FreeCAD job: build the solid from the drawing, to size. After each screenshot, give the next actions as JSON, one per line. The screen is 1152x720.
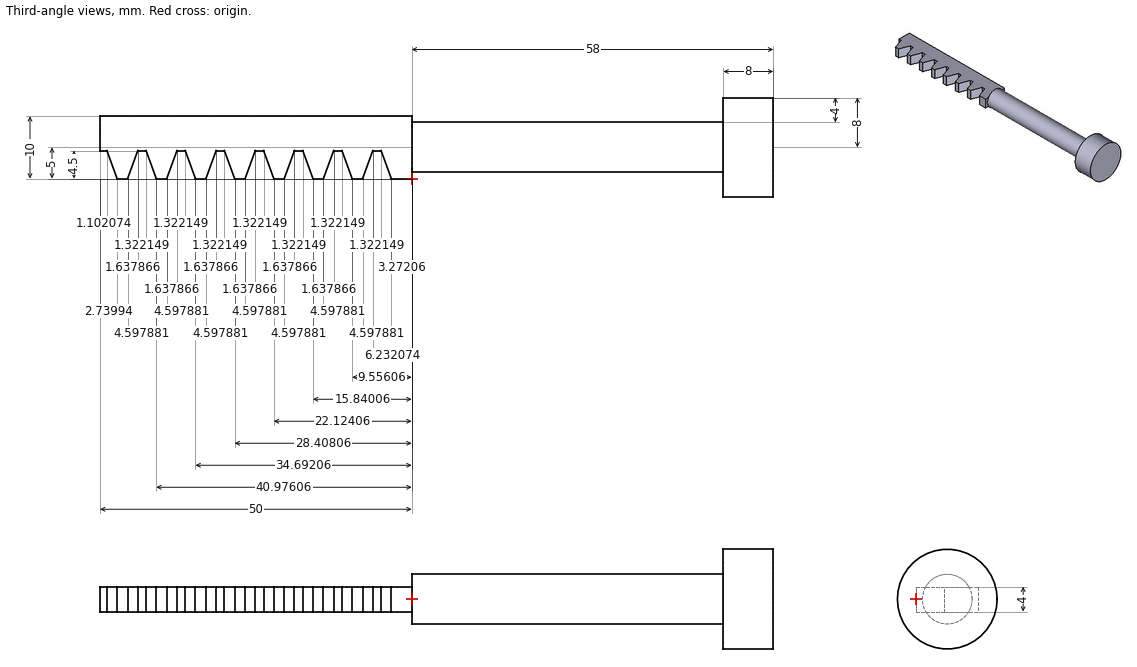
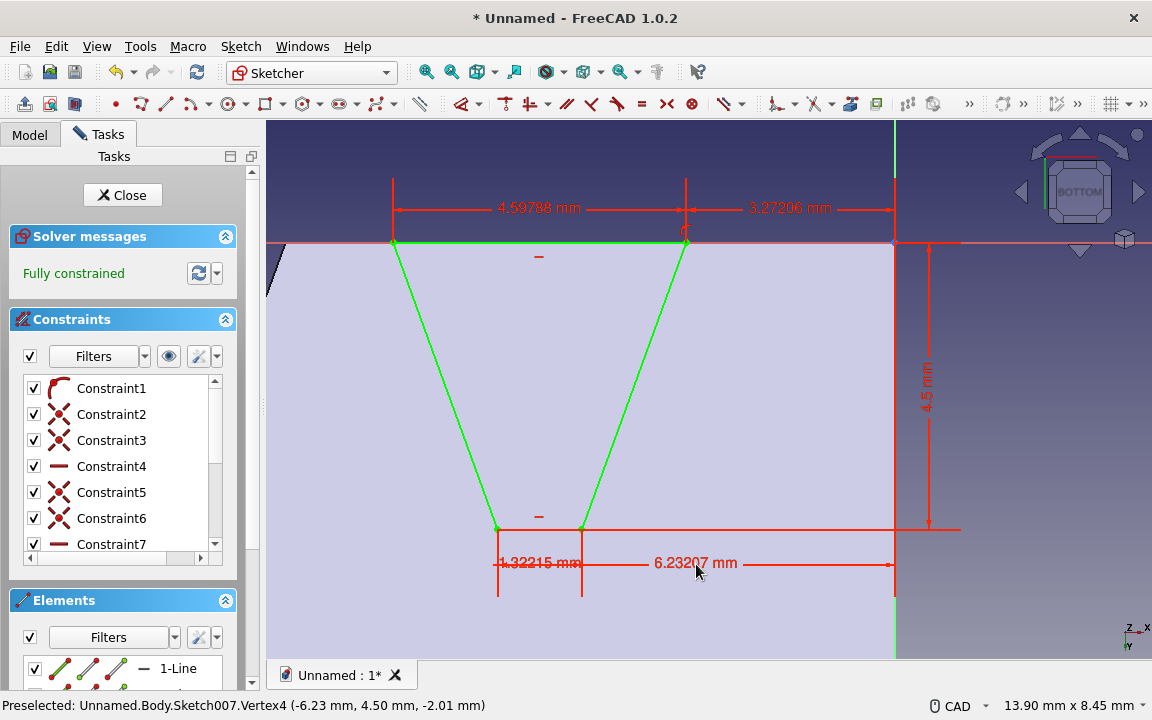
{"action": "left_click", "coordinate": [123, 195]}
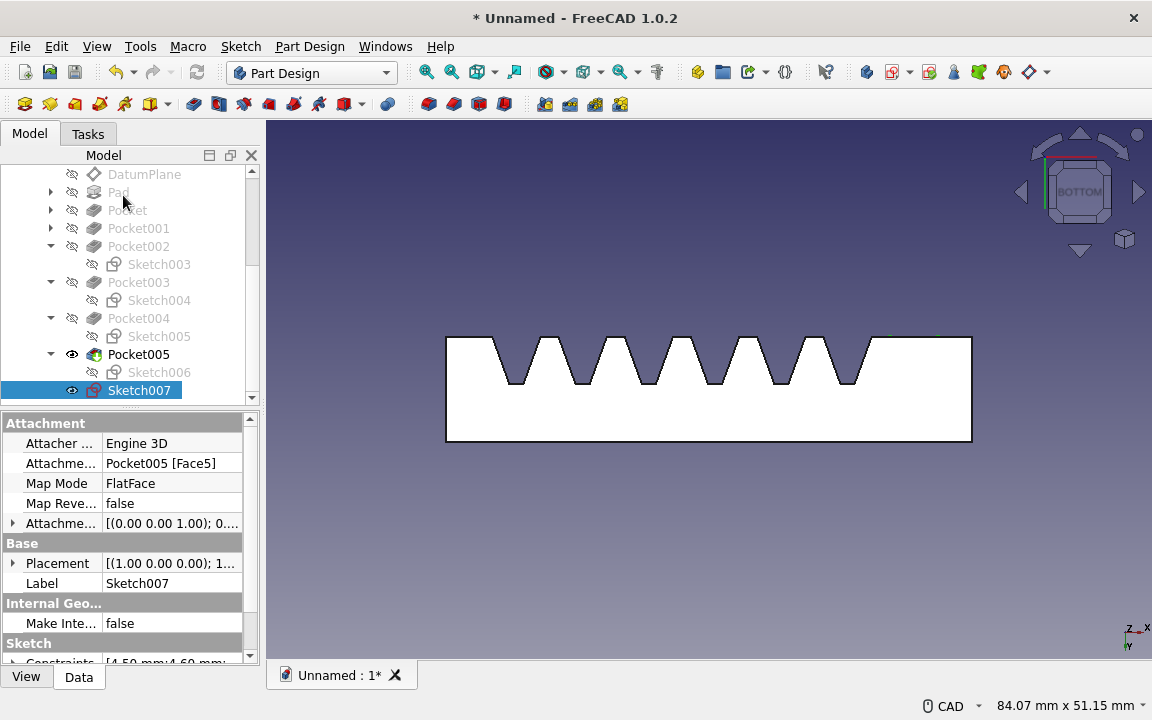
{"action": "left_click", "coordinate": [194, 104]}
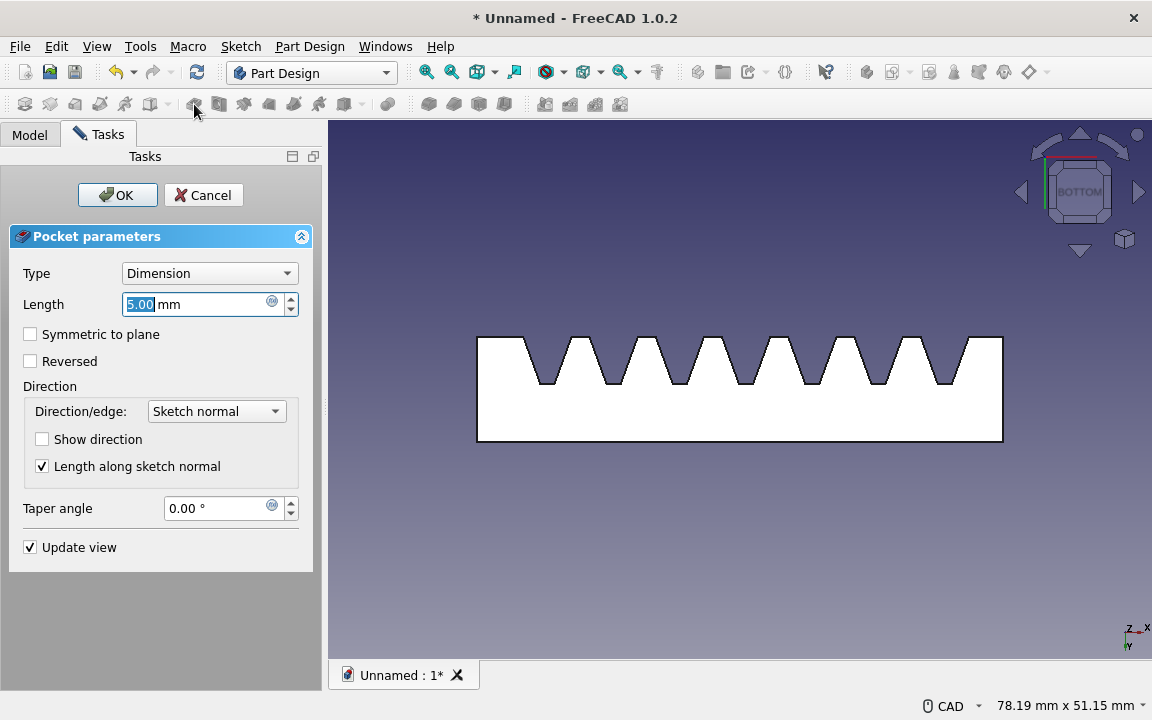
{"action": "left_click", "coordinate": [210, 274]}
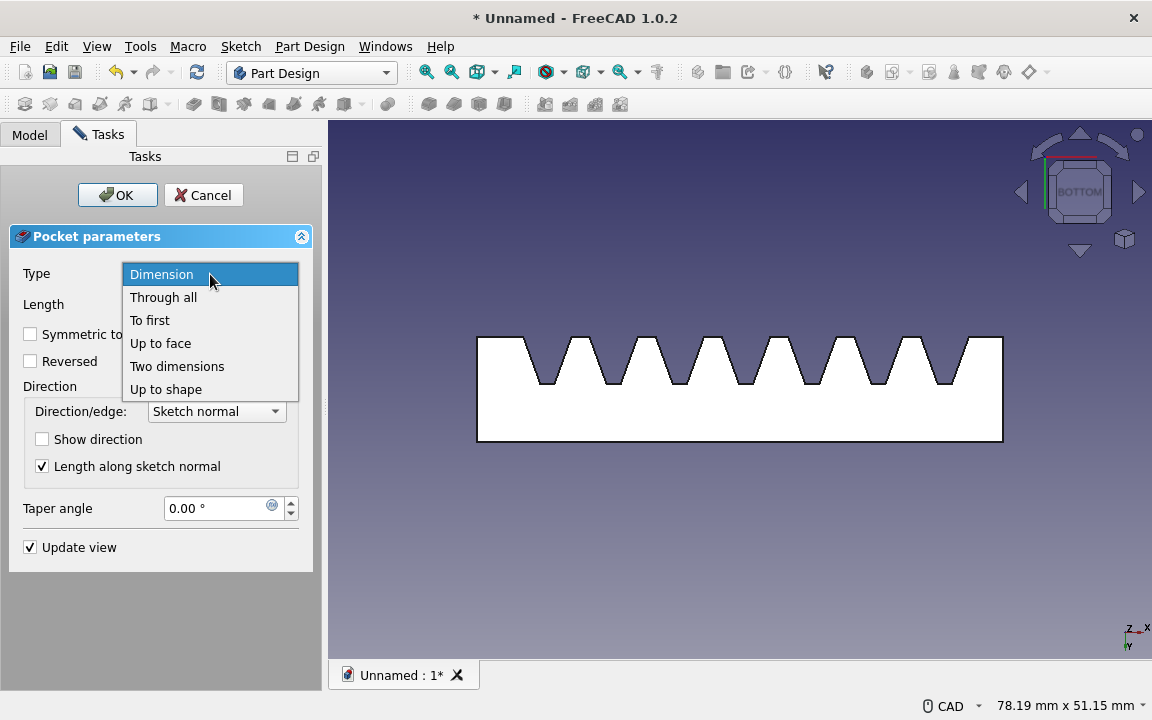
{"action": "left_click", "coordinate": [208, 298]}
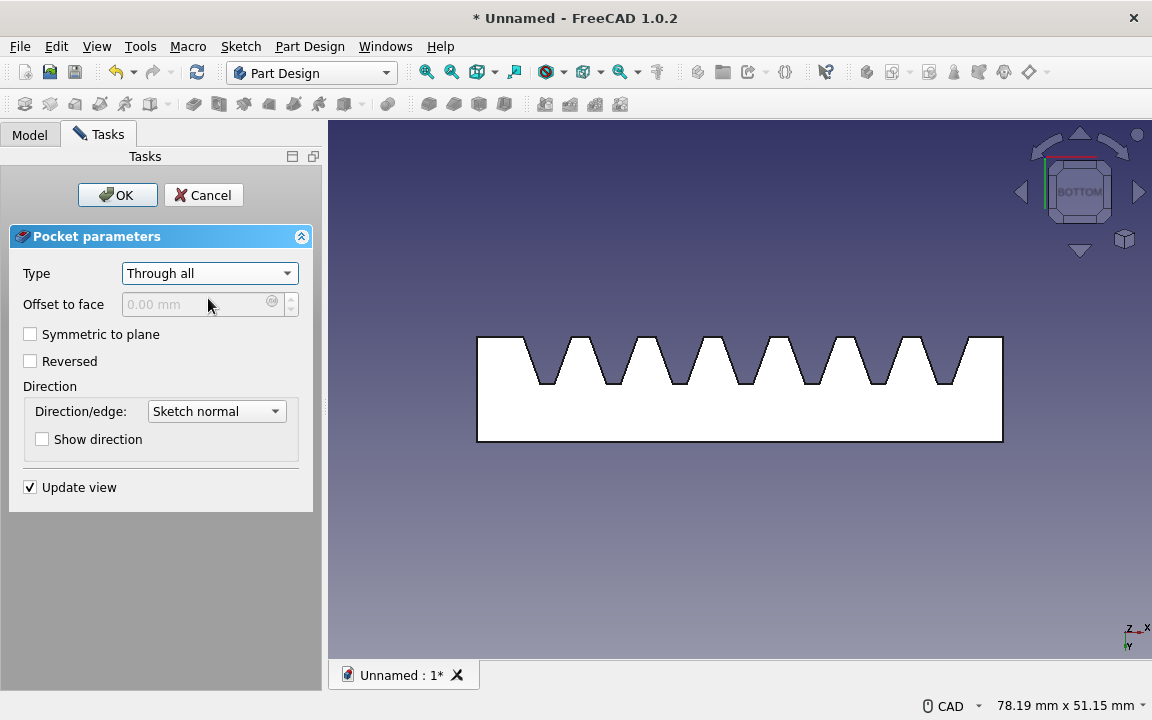
{"action": "left_click", "coordinate": [118, 195]}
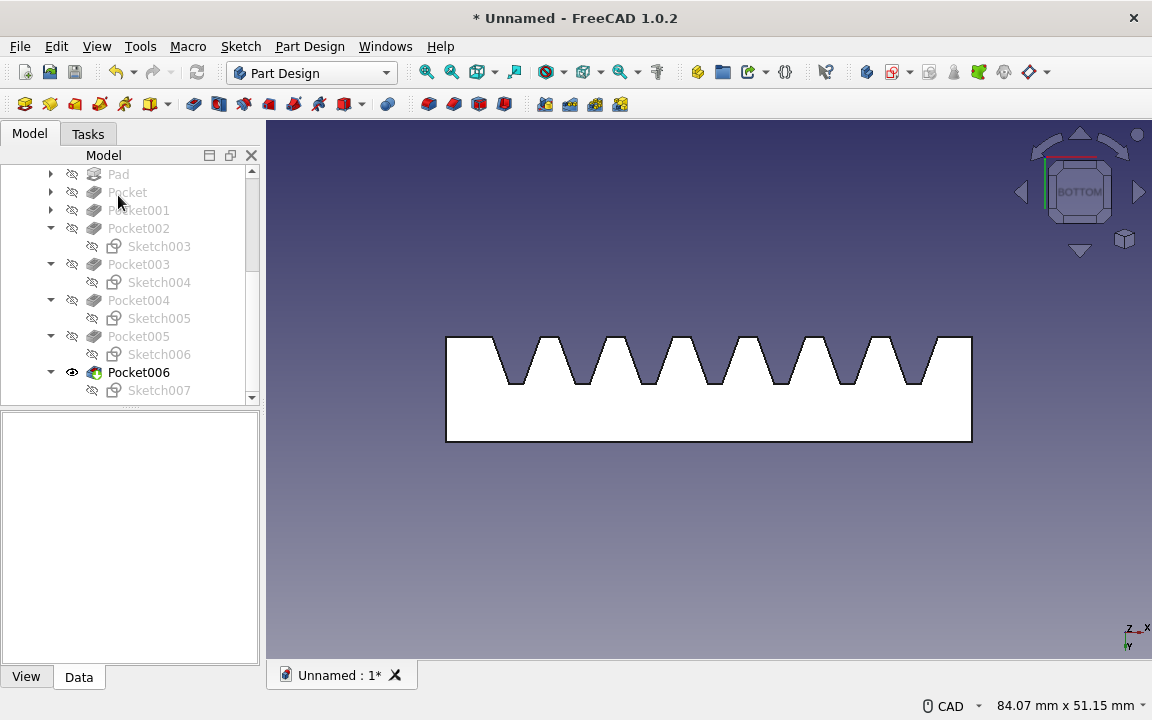
{"action": "left_click", "coordinate": [483, 404]}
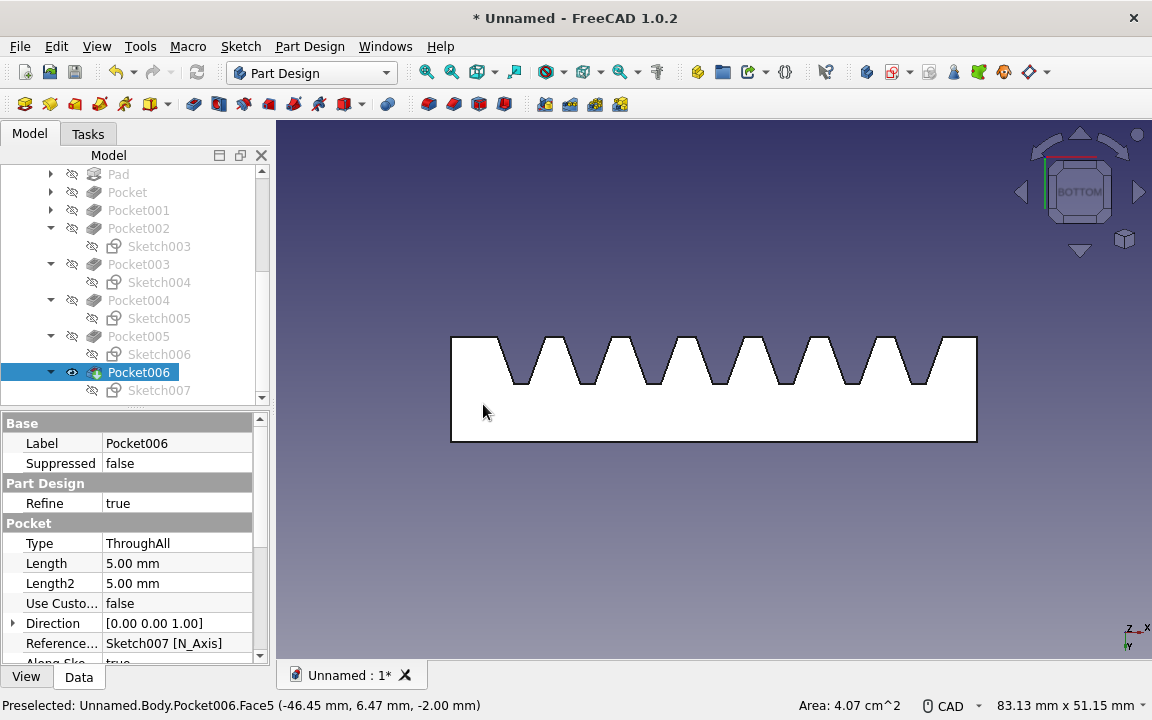
{"action": "left_click", "coordinate": [892, 72]}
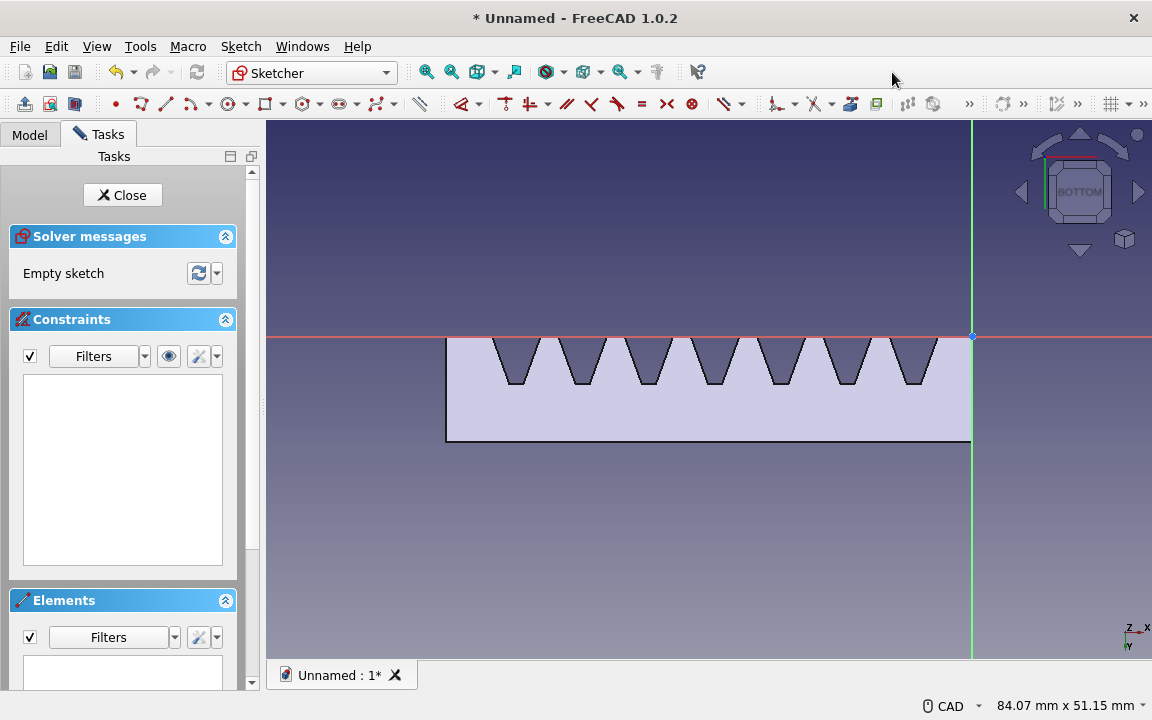
{"action": "scroll", "coordinate": [432, 356], "scroll_direction": "up", "scroll_amount": 10}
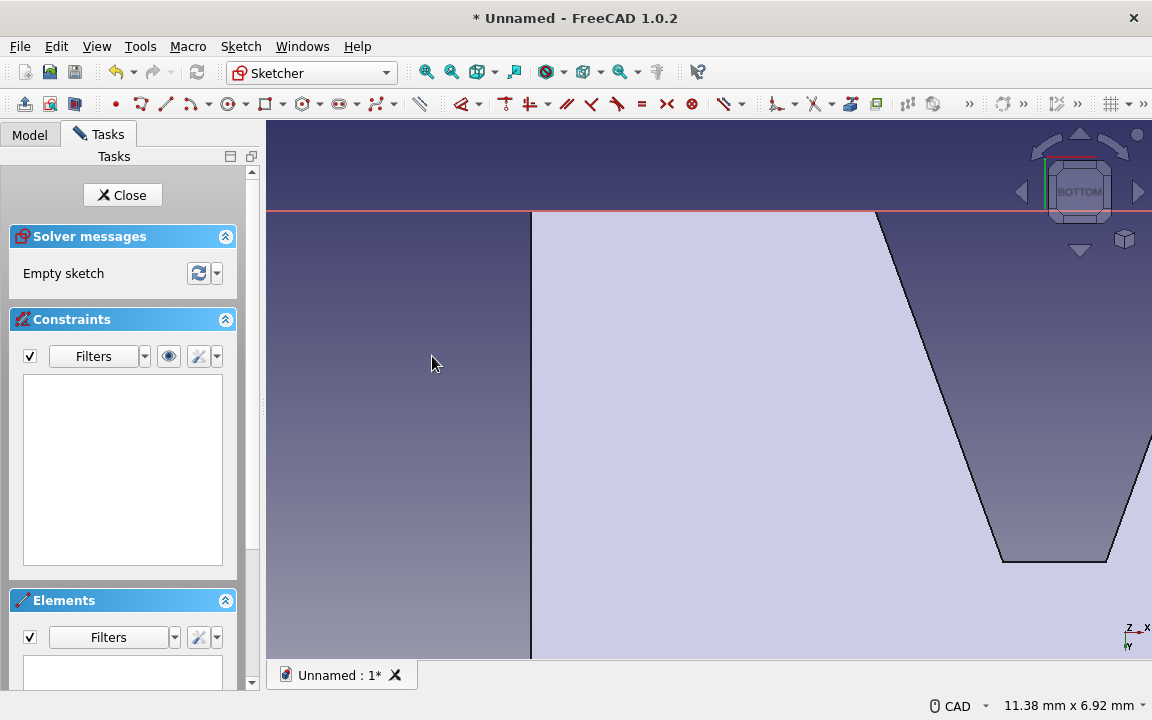
{"action": "left_click", "coordinate": [141, 104]}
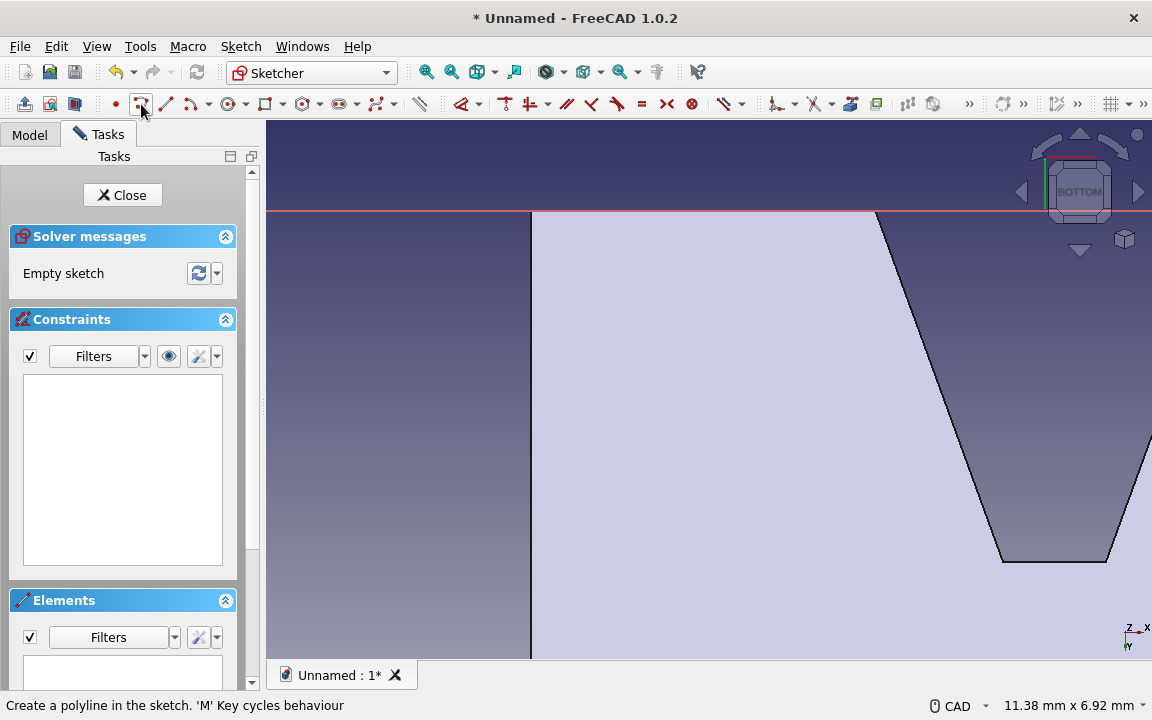
{"action": "left_click", "coordinate": [744, 211]}
{"action": "left_click", "coordinate": [531, 220]}
{"action": "left_click", "coordinate": [531, 562]}
{"action": "left_click", "coordinate": [617, 562]}
{"action": "left_click", "coordinate": [744, 211]}
{"action": "key", "text": "Escape"}
{"action": "key", "text": "Escape"}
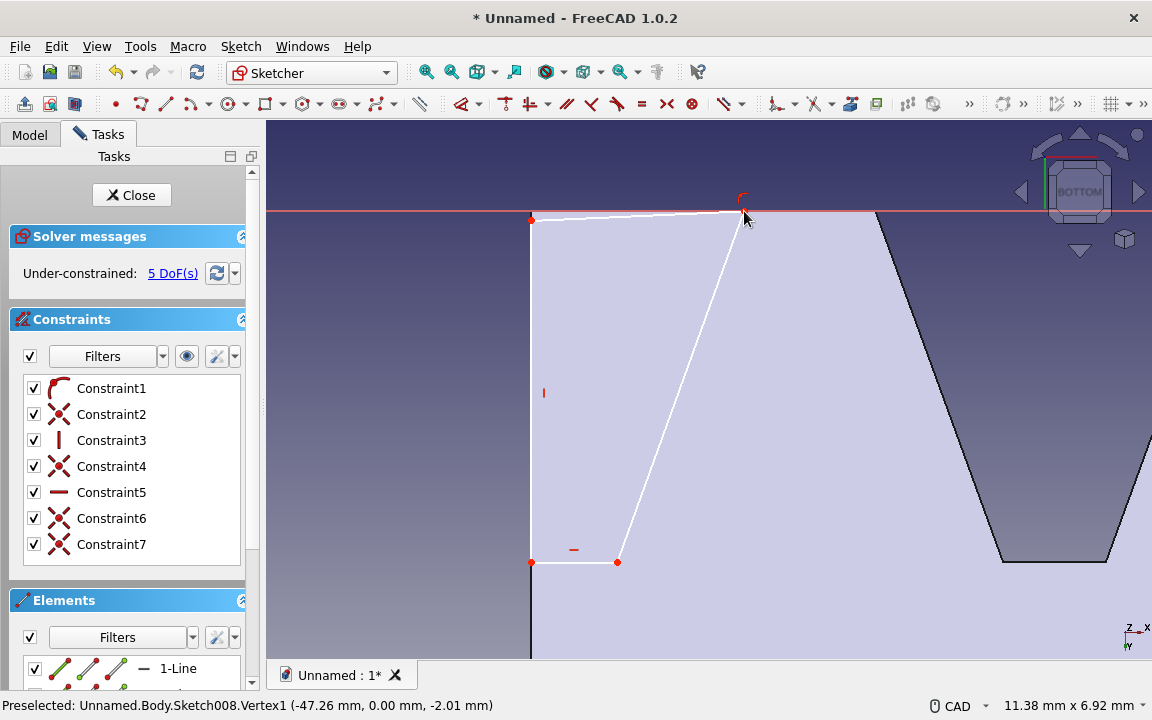
{"action": "left_click", "coordinate": [680, 214]}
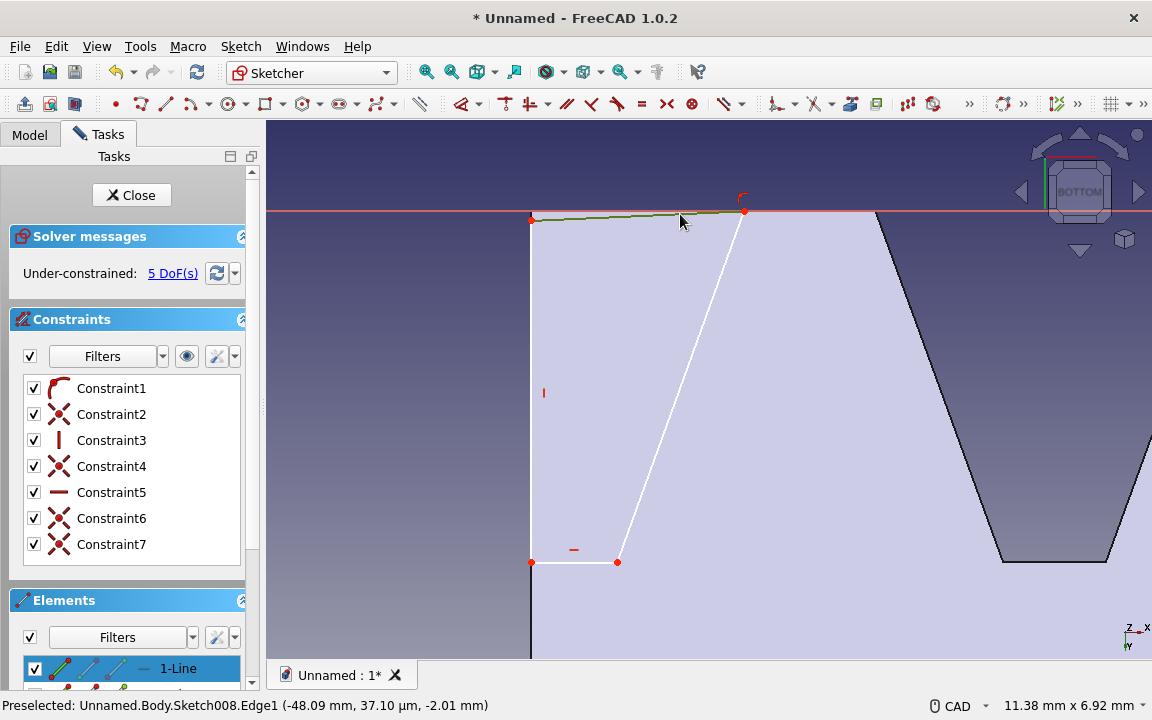
{"action": "left_click", "coordinate": [548, 104]}